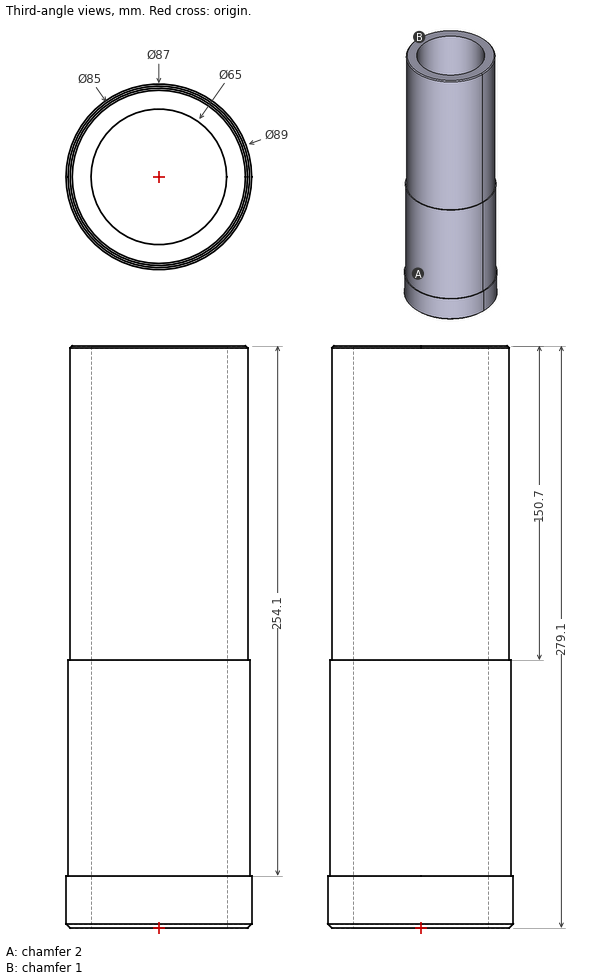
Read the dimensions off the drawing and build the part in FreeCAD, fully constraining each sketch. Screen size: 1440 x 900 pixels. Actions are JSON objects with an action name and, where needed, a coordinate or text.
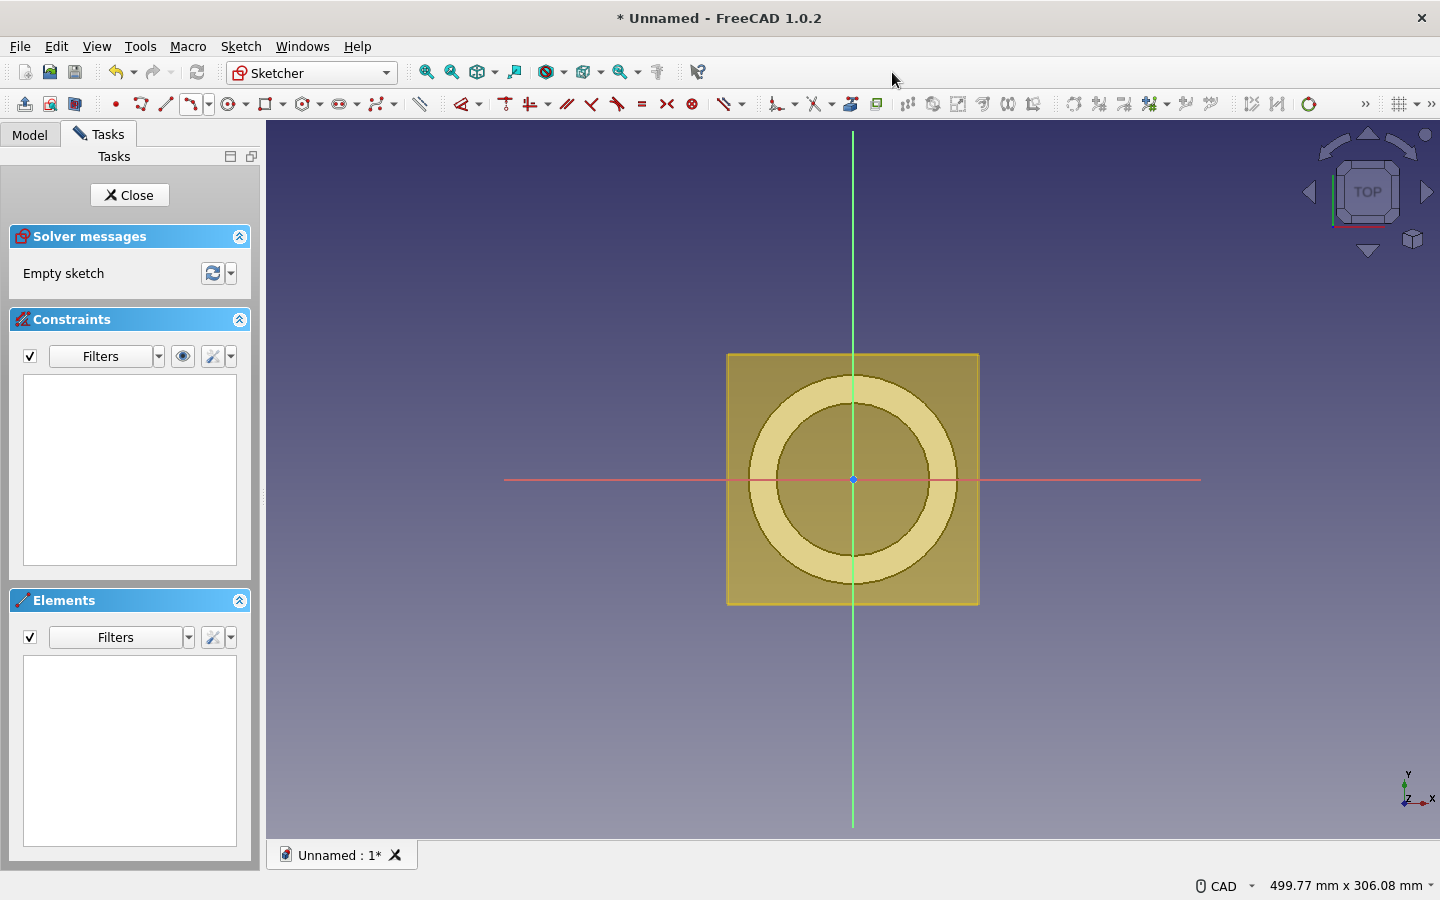
{"action": "scroll", "coordinate": [909, 480], "scroll_direction": "up", "scroll_amount": 4}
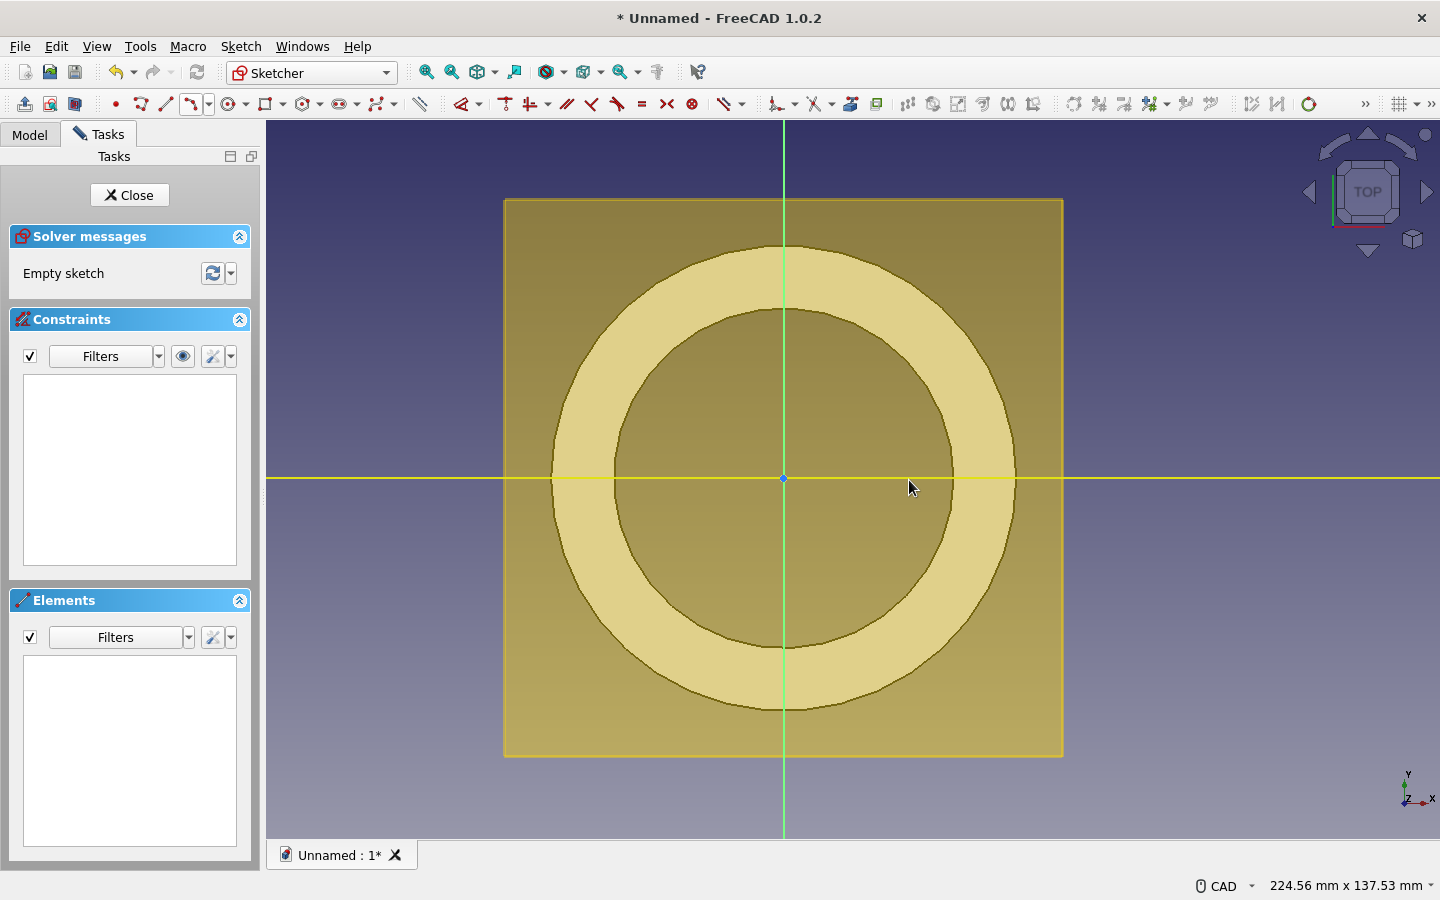
{"action": "left_click", "coordinate": [228, 104]}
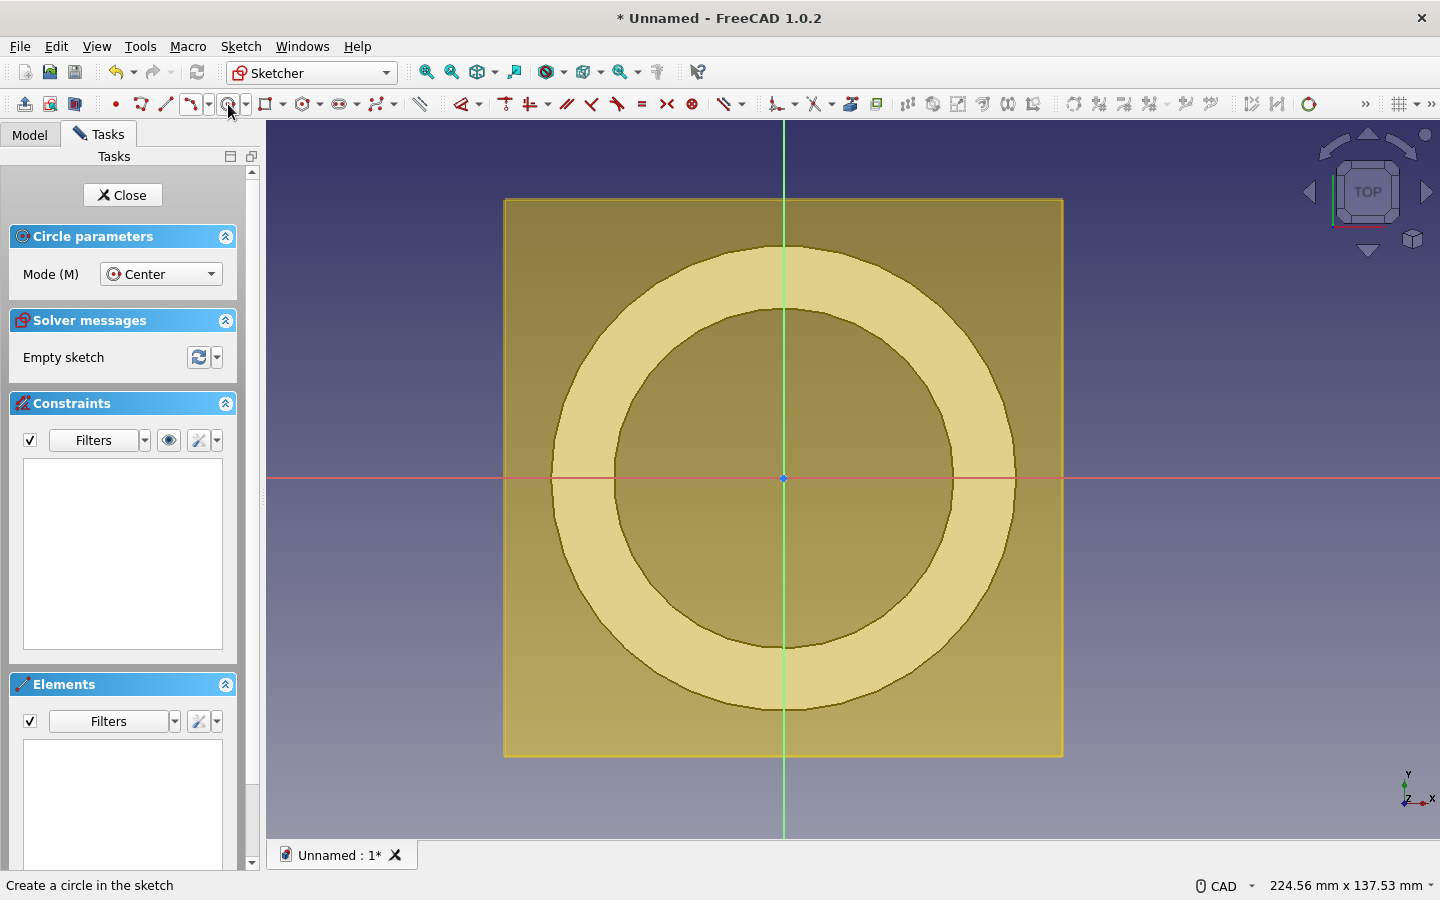
{"action": "left_click", "coordinate": [784, 478]}
{"action": "mouse_move", "coordinate": [948, 314]}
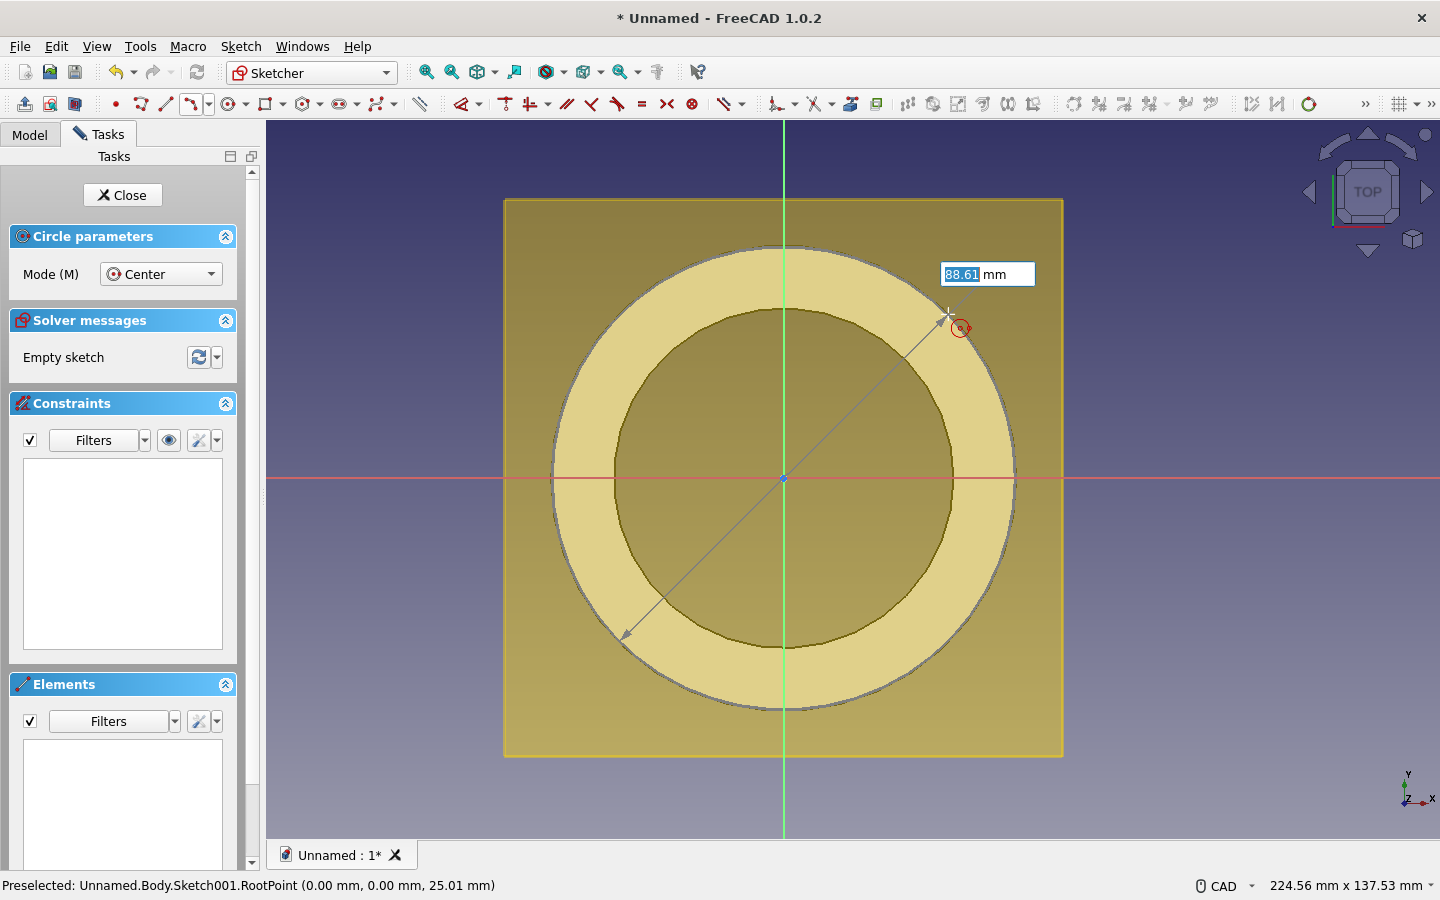
{"action": "type", "text": "89"}
{"action": "key", "text": "Return"}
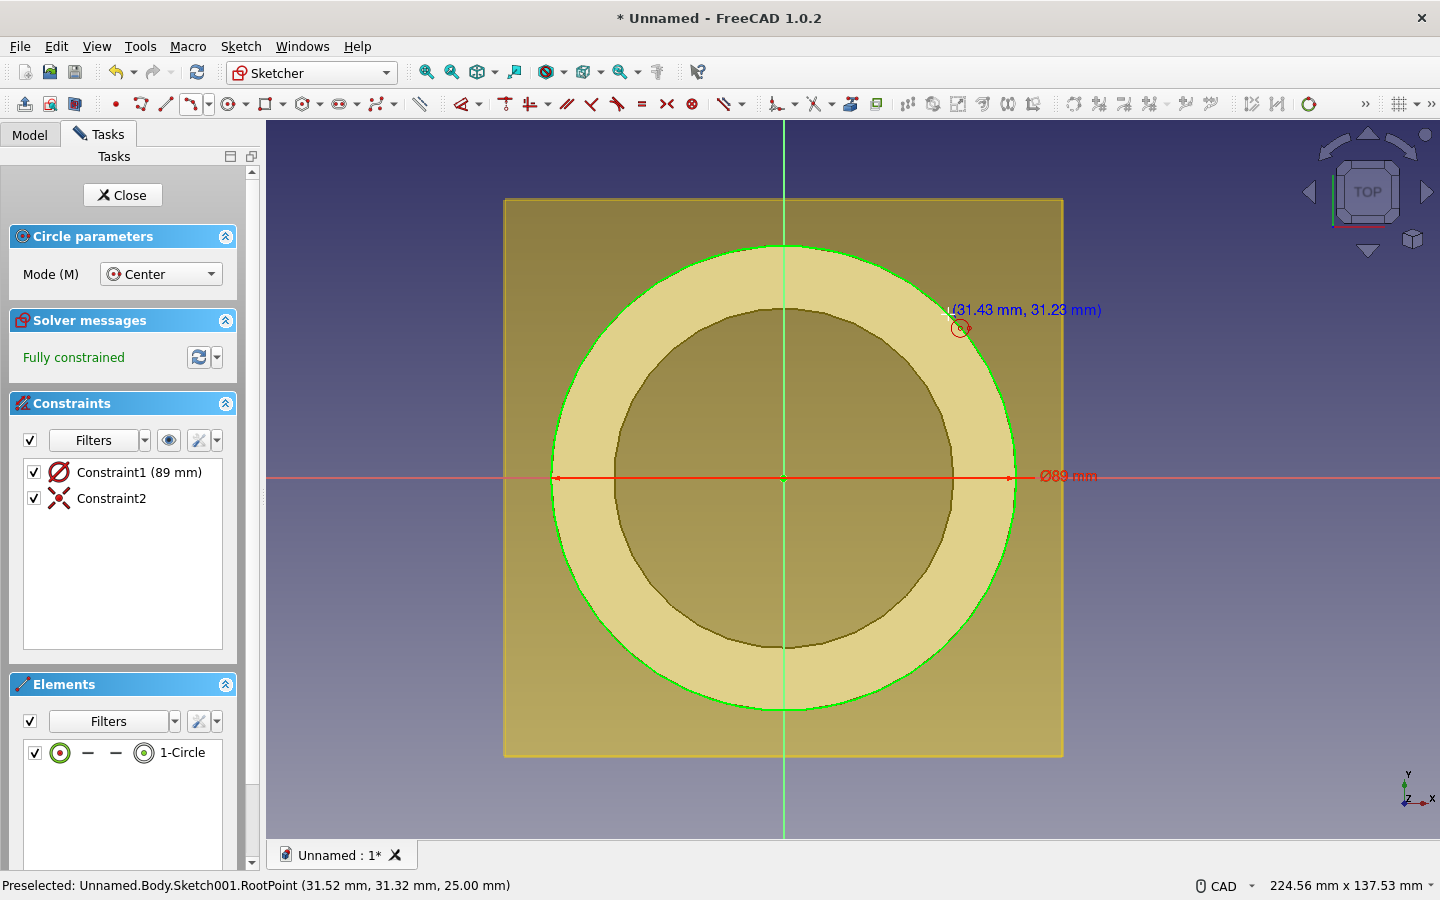
{"action": "left_click", "coordinate": [784, 478]}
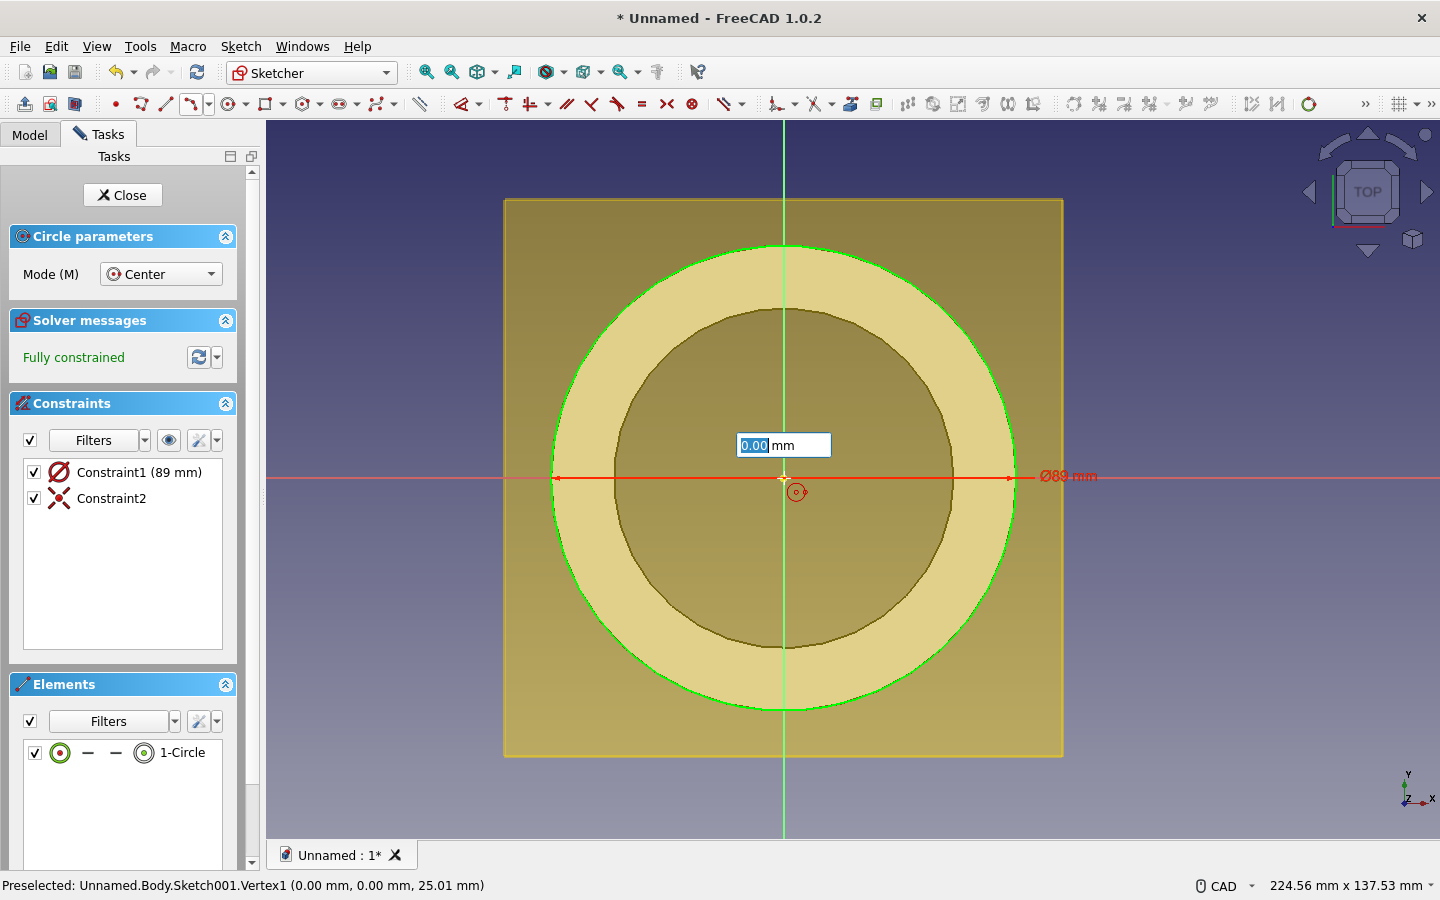
{"action": "scroll", "coordinate": [945, 317], "scroll_direction": "up", "scroll_amount": 6}
{"action": "mouse_move", "coordinate": [942, 318]}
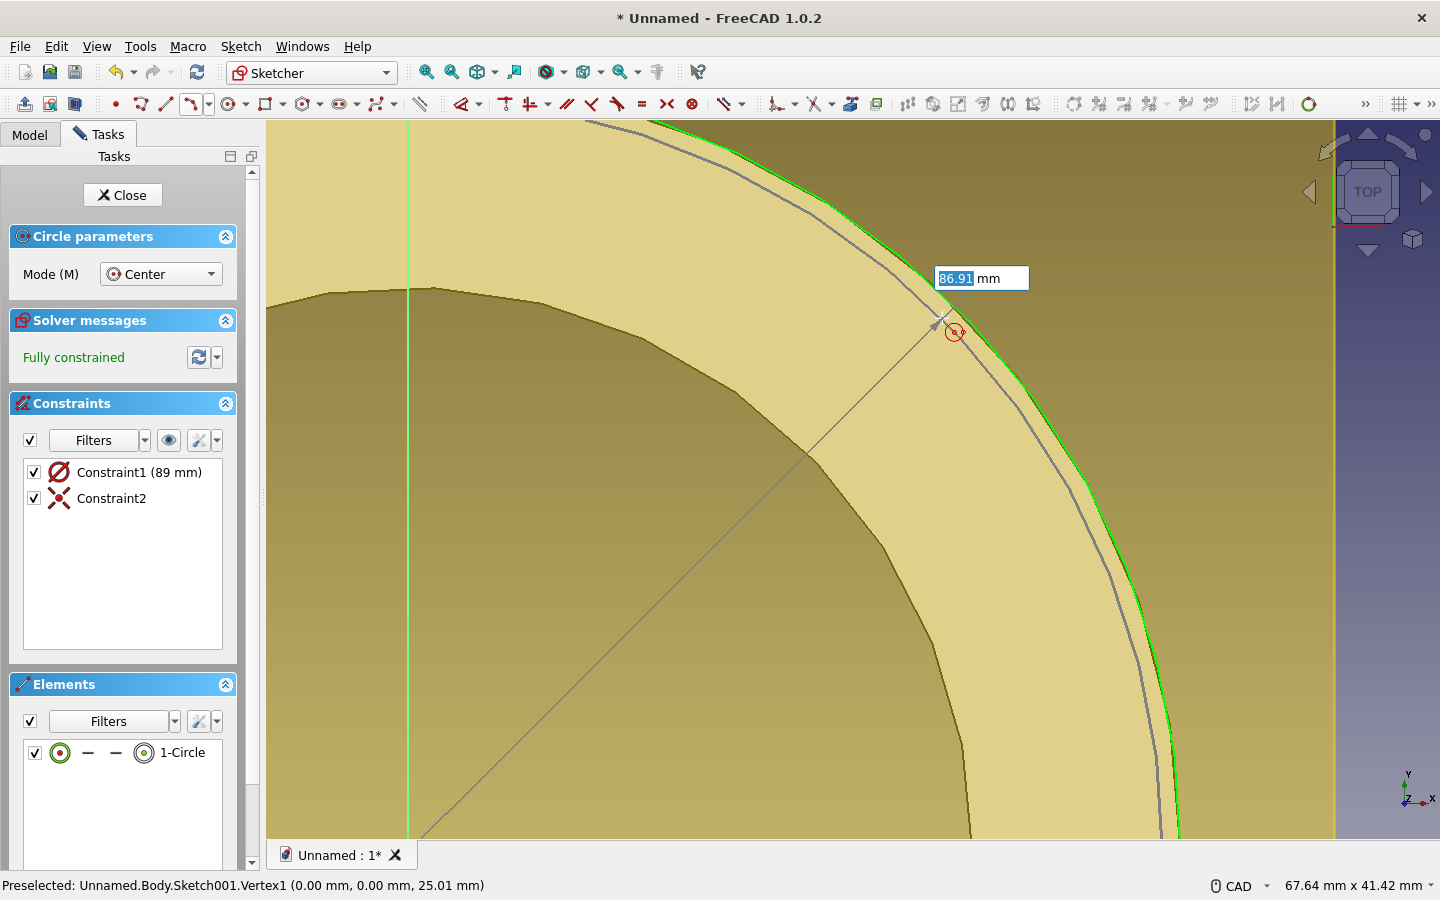
{"action": "type", "text": "87"}
{"action": "key", "text": "Return"}
{"action": "key", "text": "Escape"}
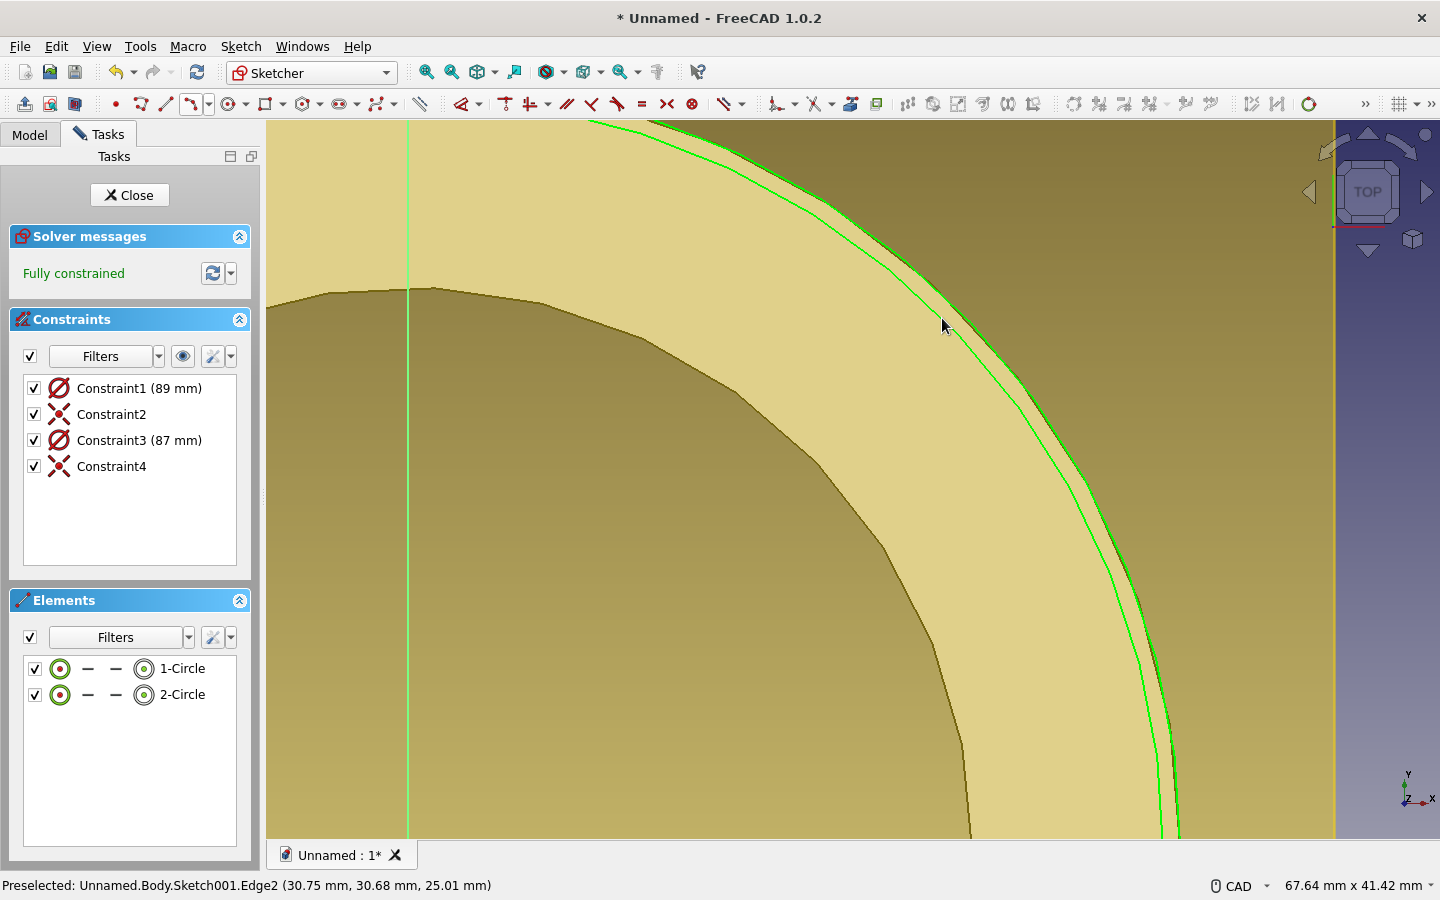
{"action": "left_click", "coordinate": [130, 195]}